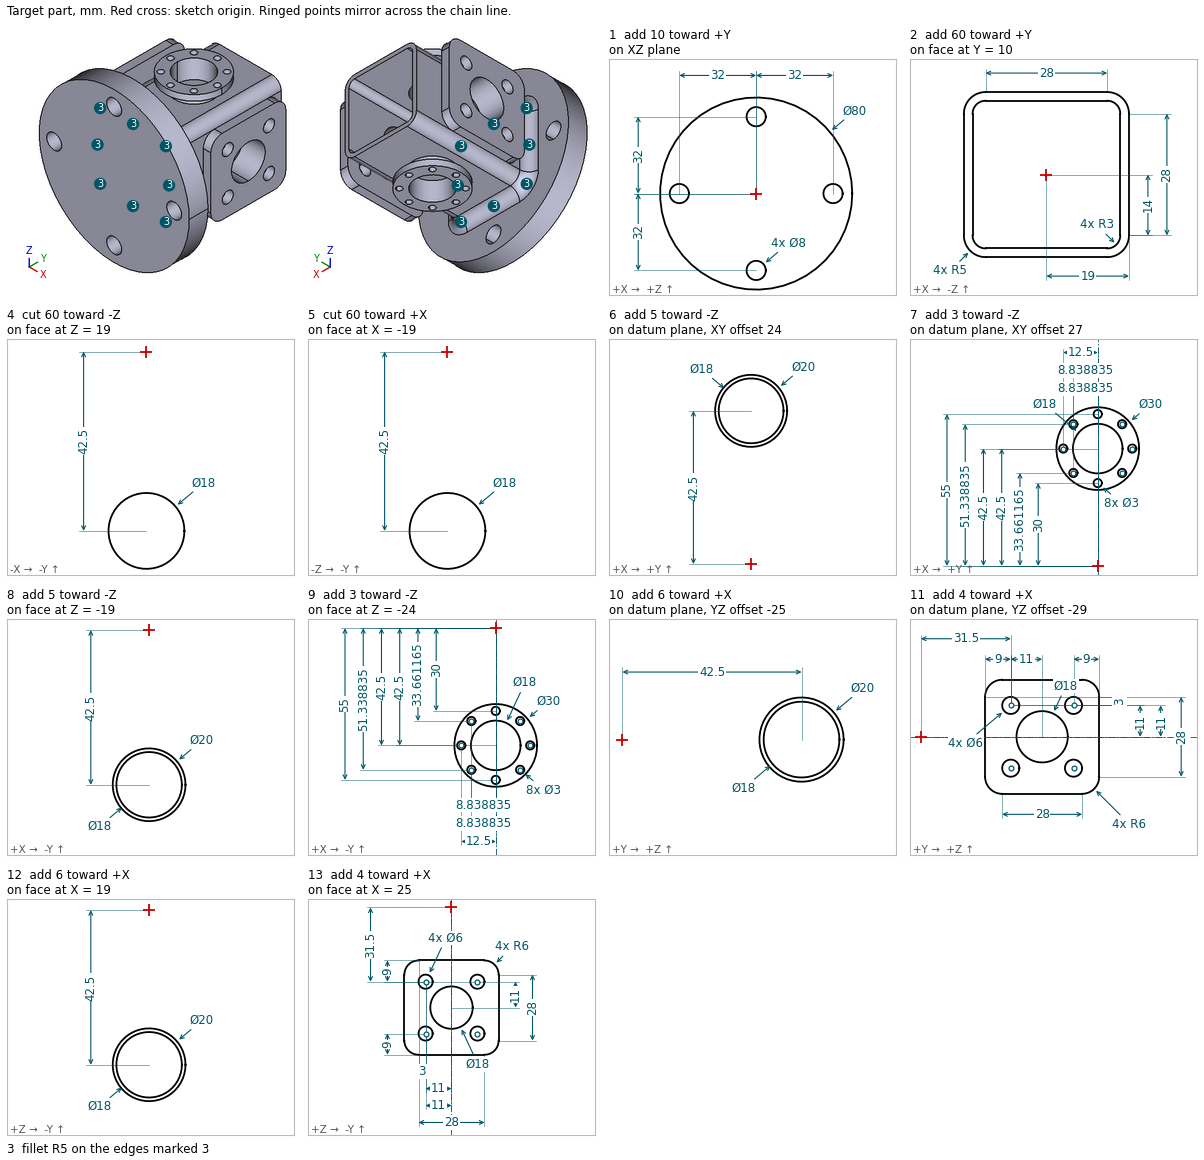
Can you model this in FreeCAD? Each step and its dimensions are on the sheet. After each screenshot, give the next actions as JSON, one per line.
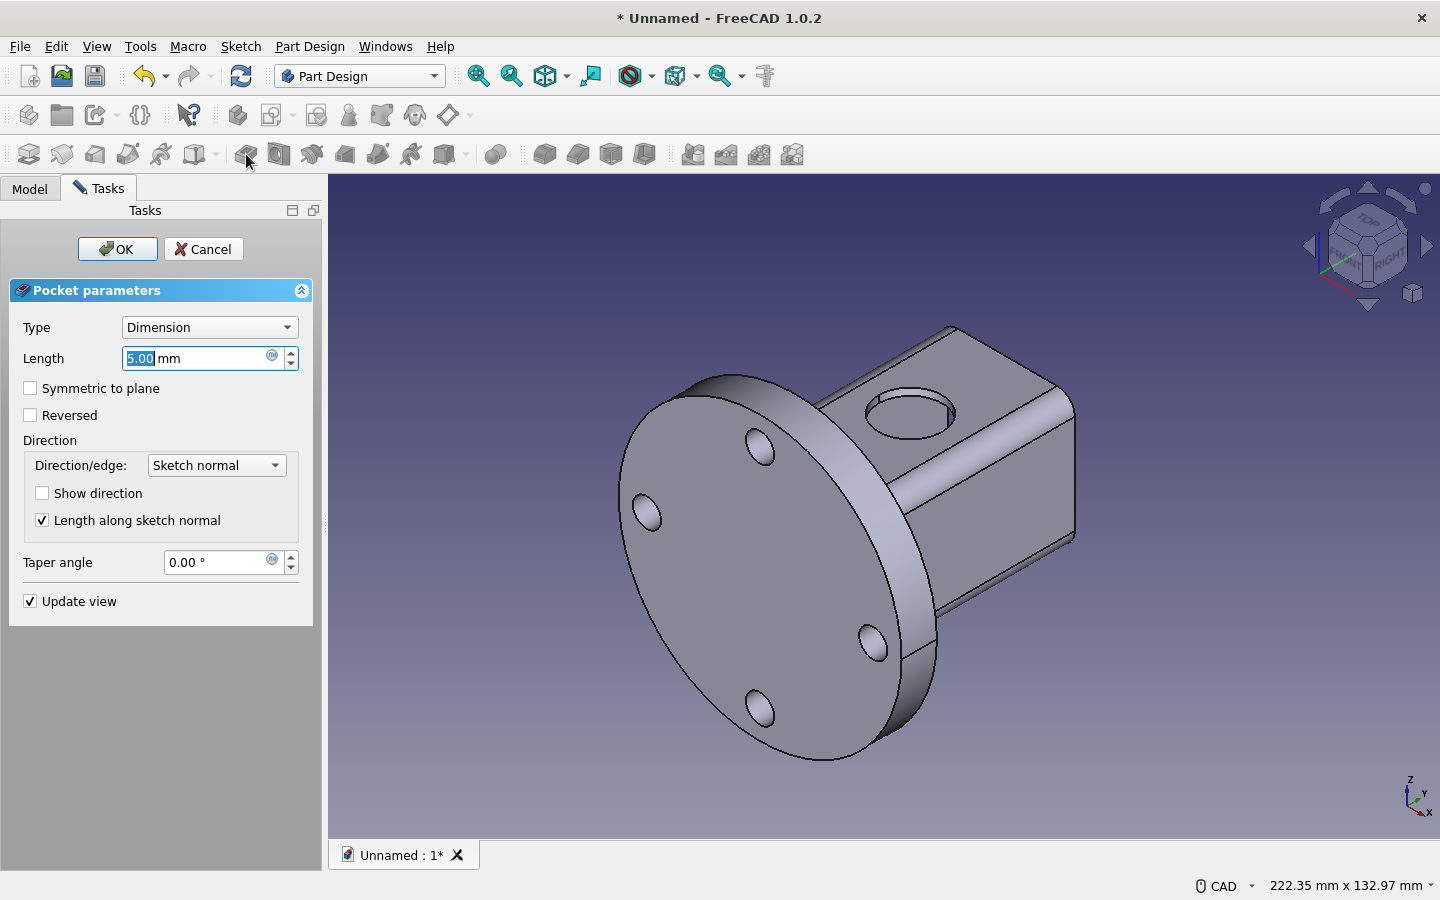
{"action": "type", "text": "60"}
{"action": "key", "text": "Tab"}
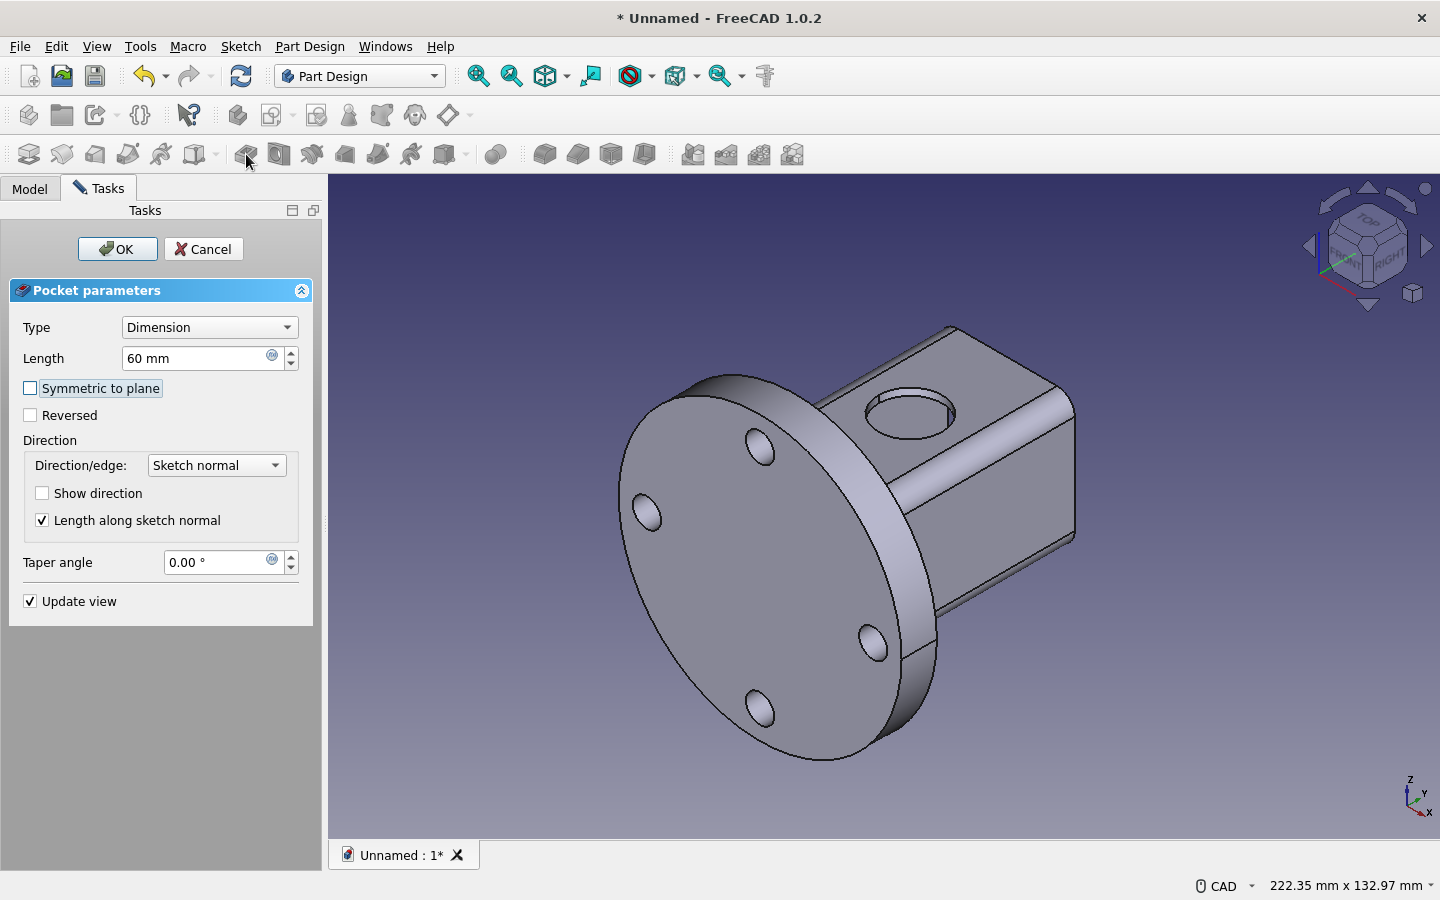
{"action": "left_click", "coordinate": [118, 249]}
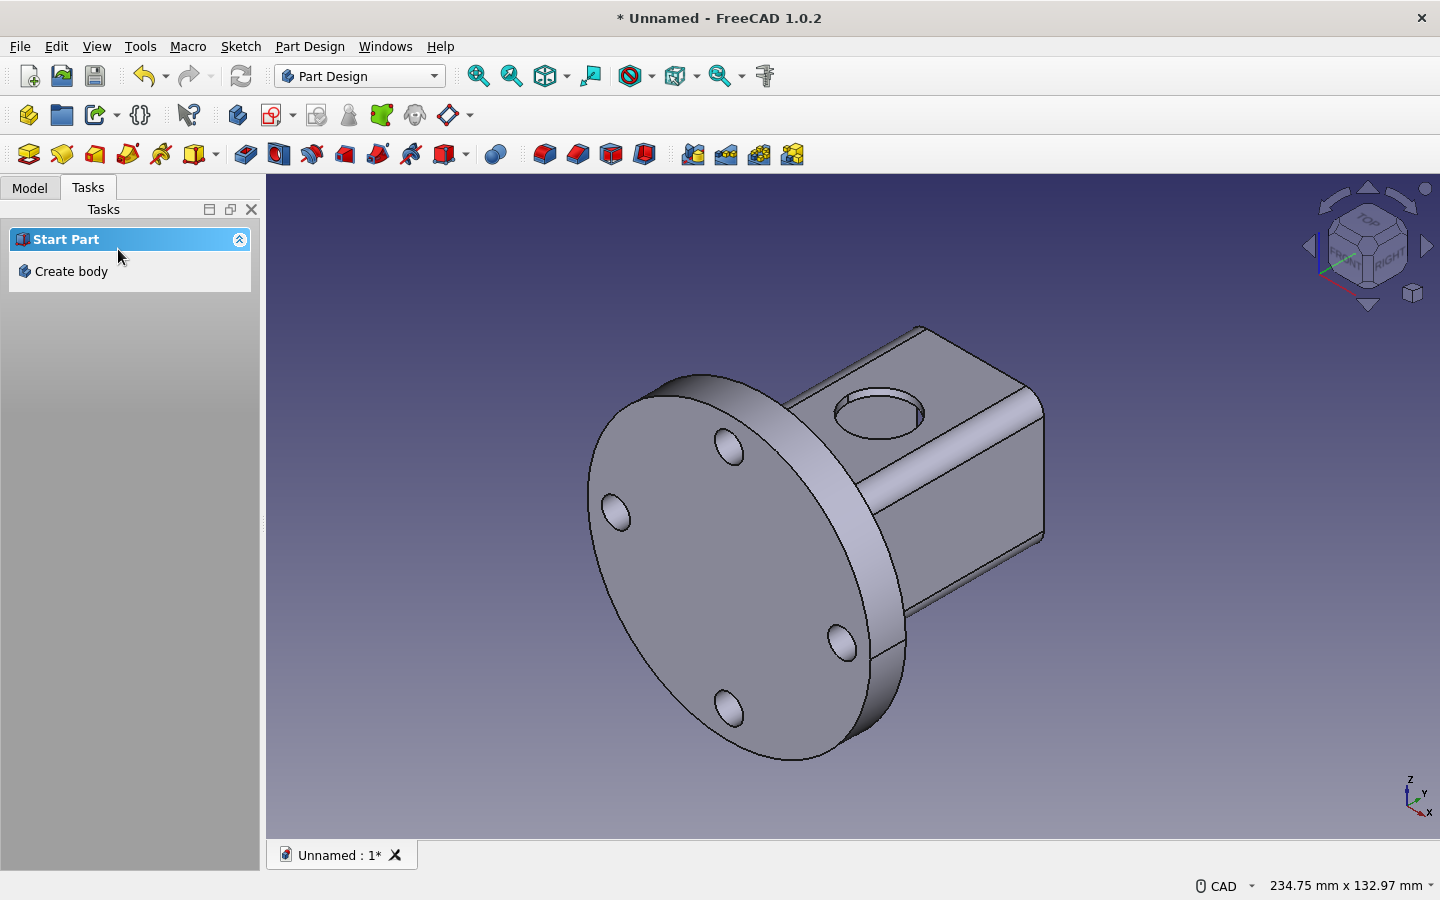
{"action": "key", "text": "6"}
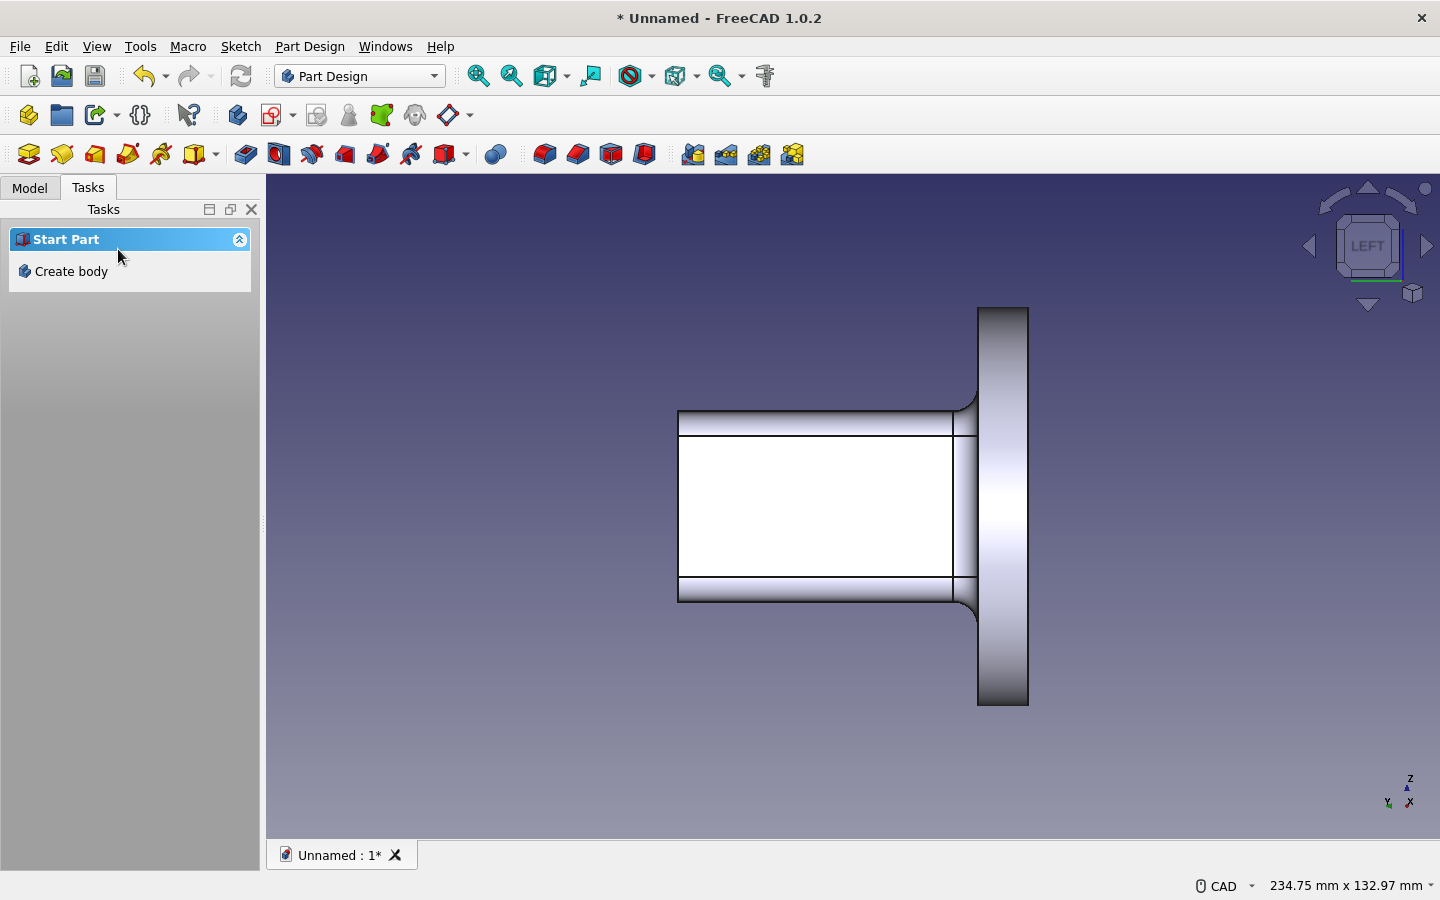
{"action": "left_click", "coordinate": [776, 505]}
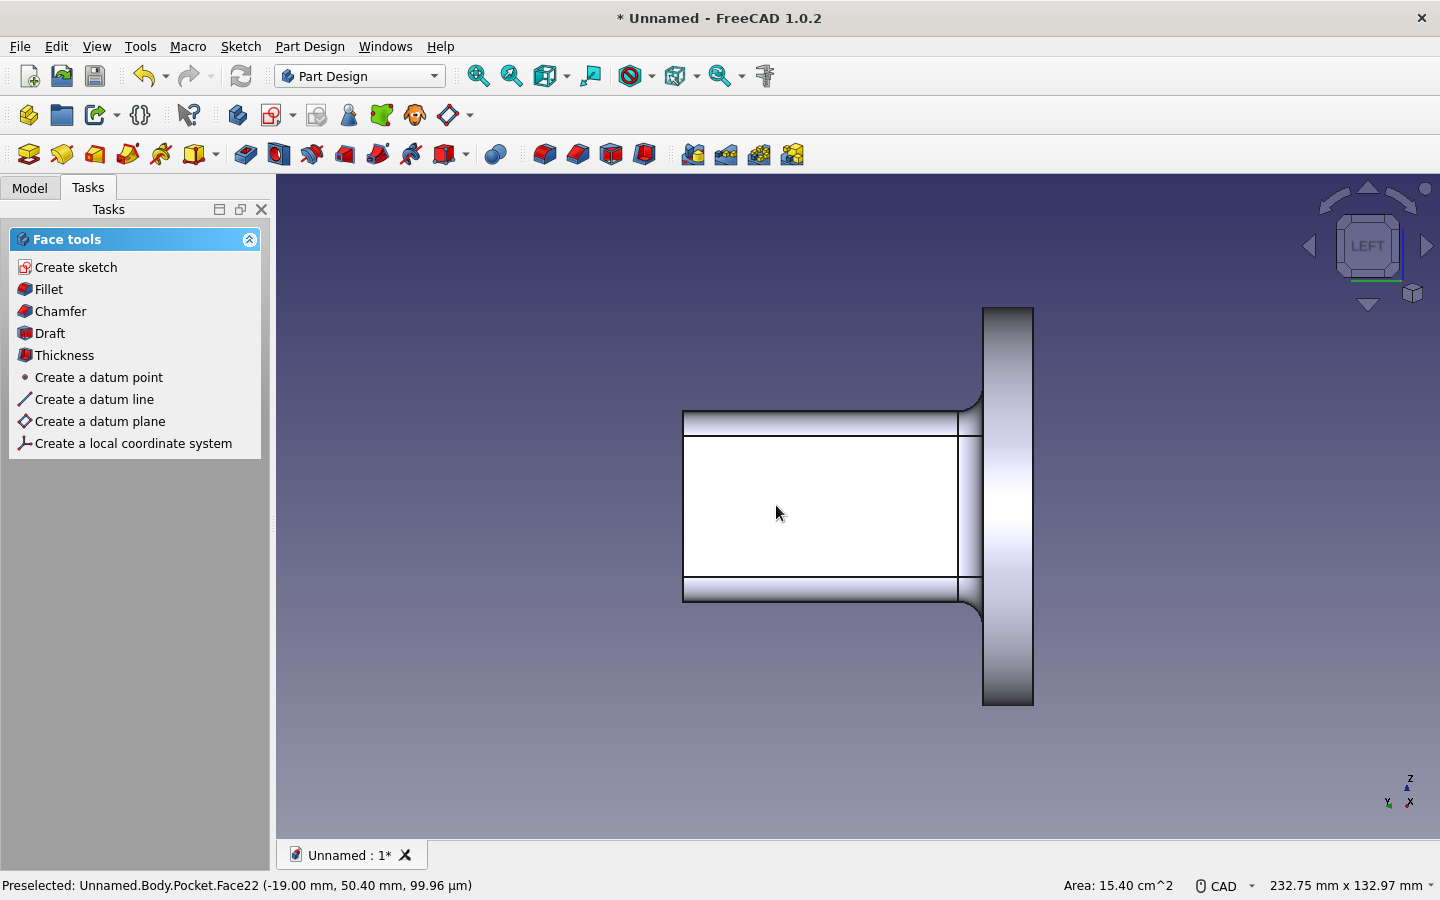
{"action": "left_click", "coordinate": [270, 116]}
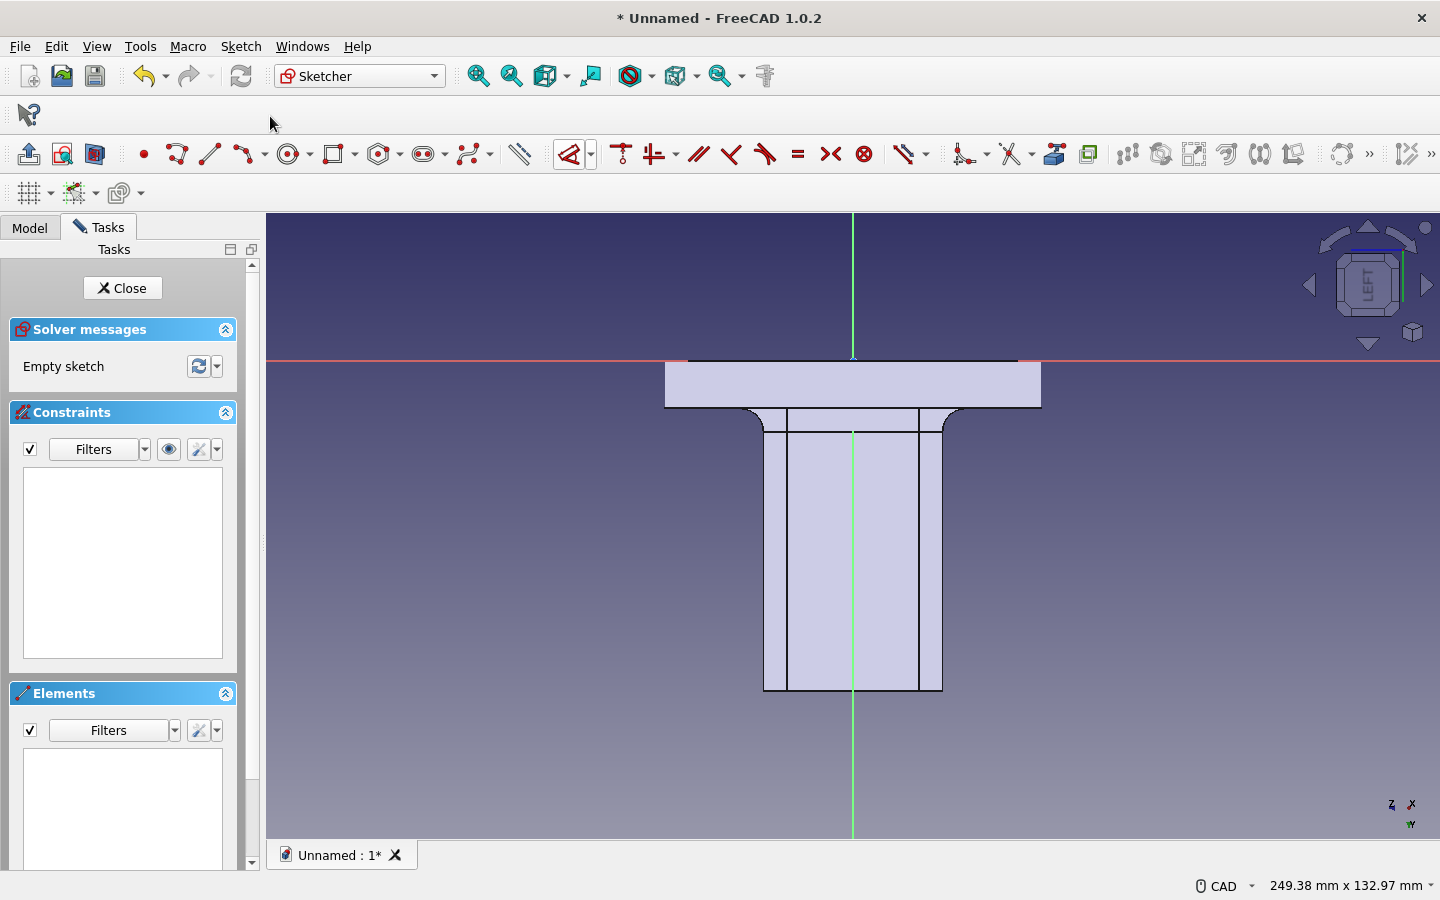
{"action": "key", "text": "q s"}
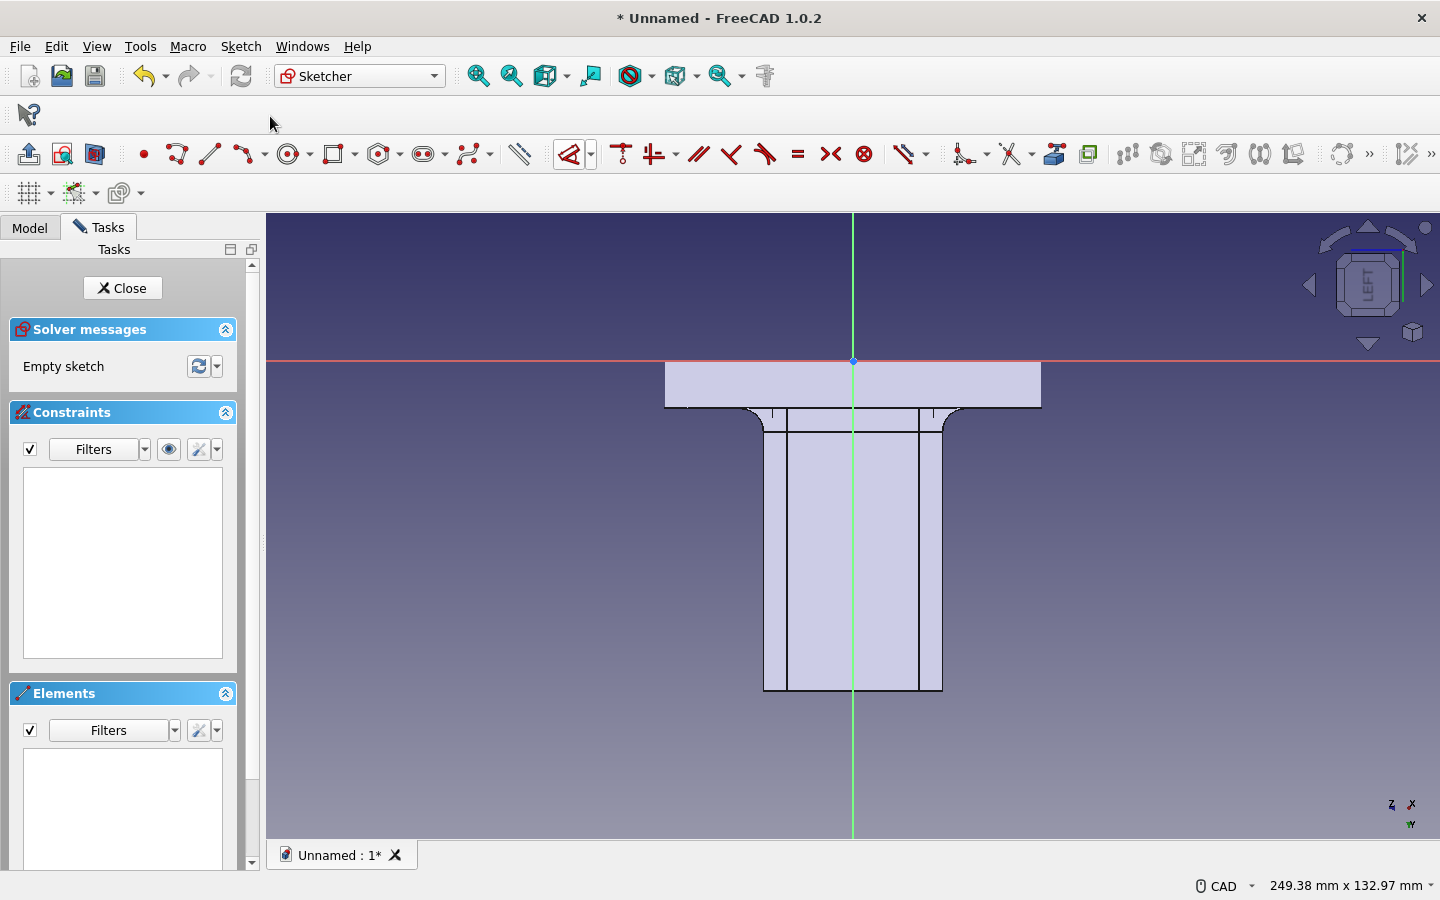
{"action": "scroll", "coordinate": [870, 570], "scroll_direction": "up", "scroll_amount": 8}